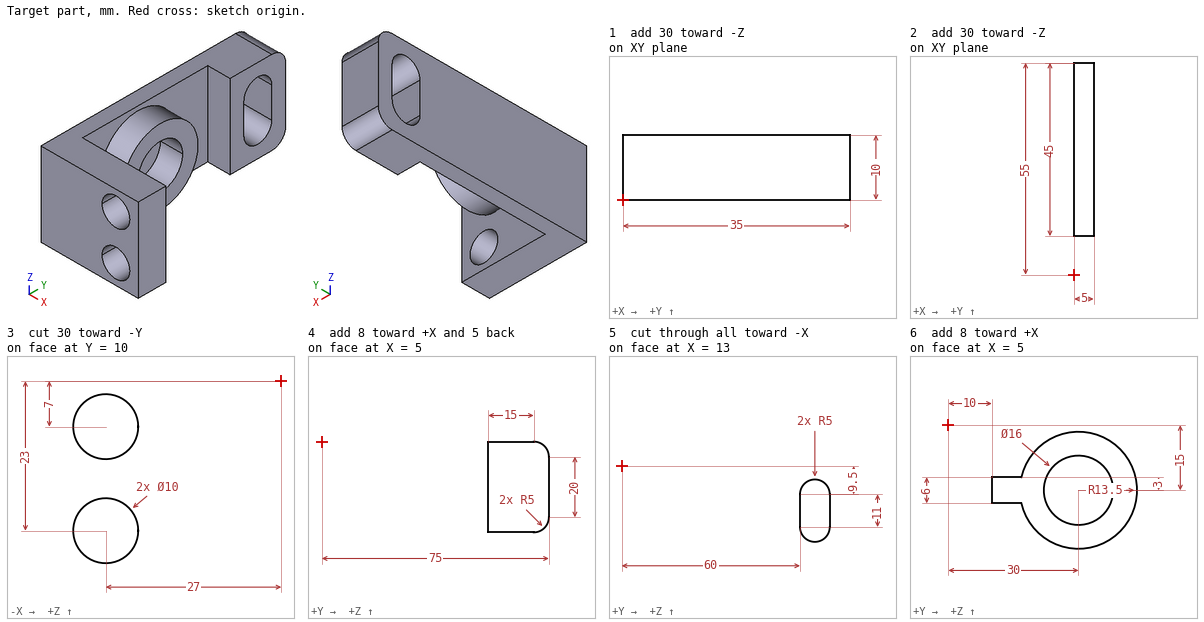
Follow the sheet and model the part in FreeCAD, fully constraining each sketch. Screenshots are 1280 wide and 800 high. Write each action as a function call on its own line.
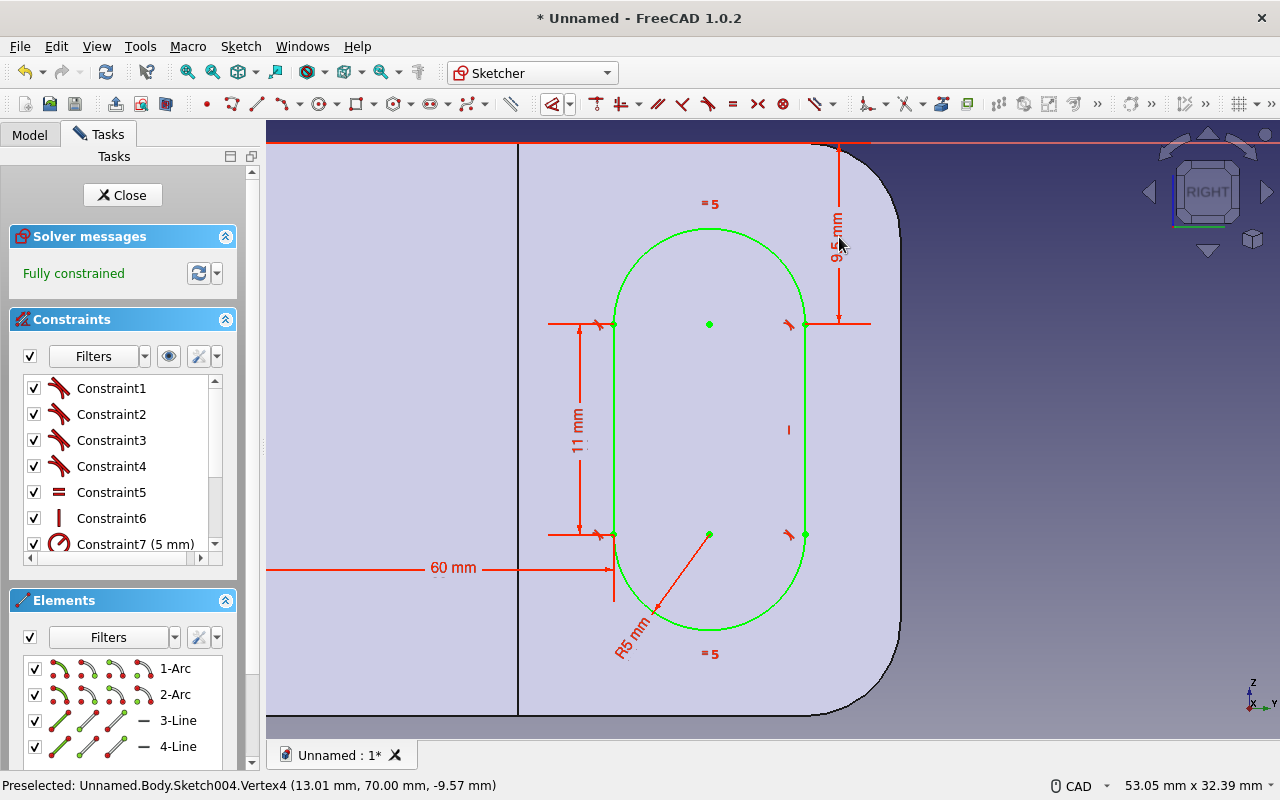
click(123, 195)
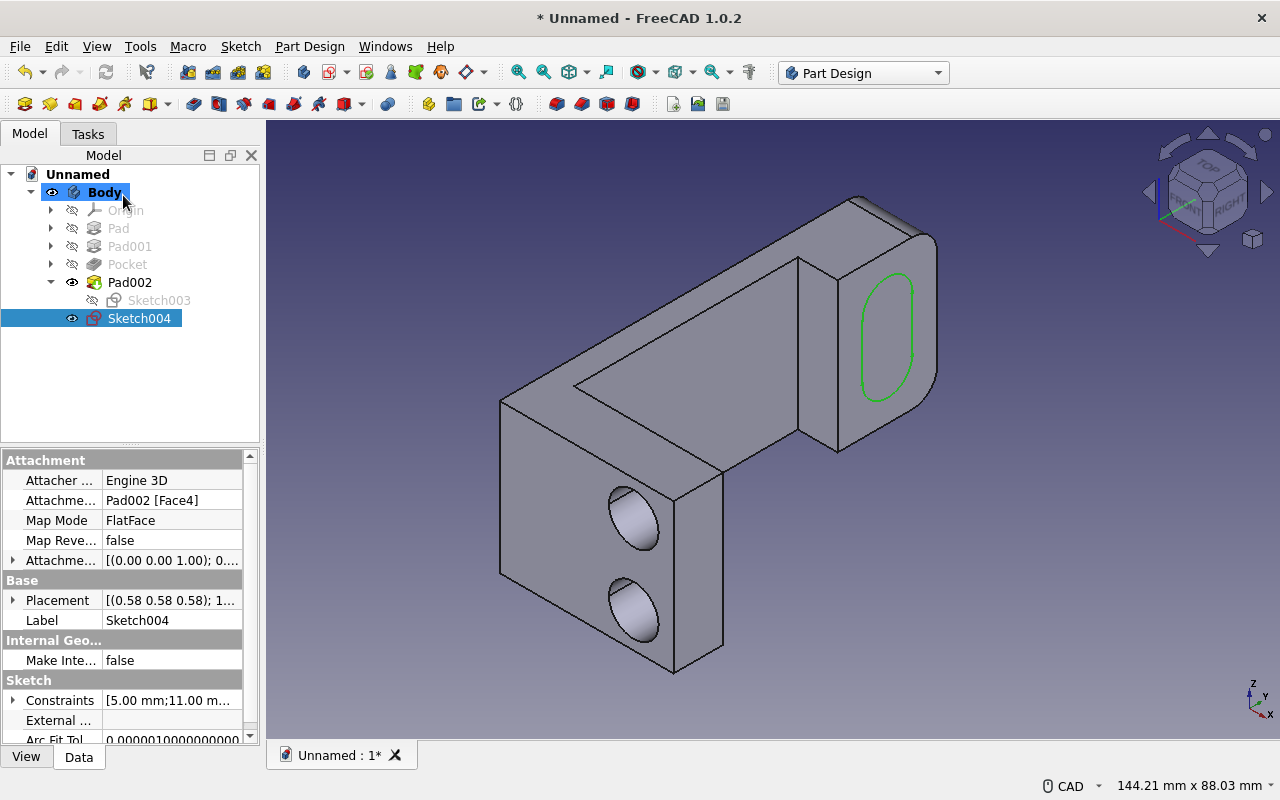
click(194, 104)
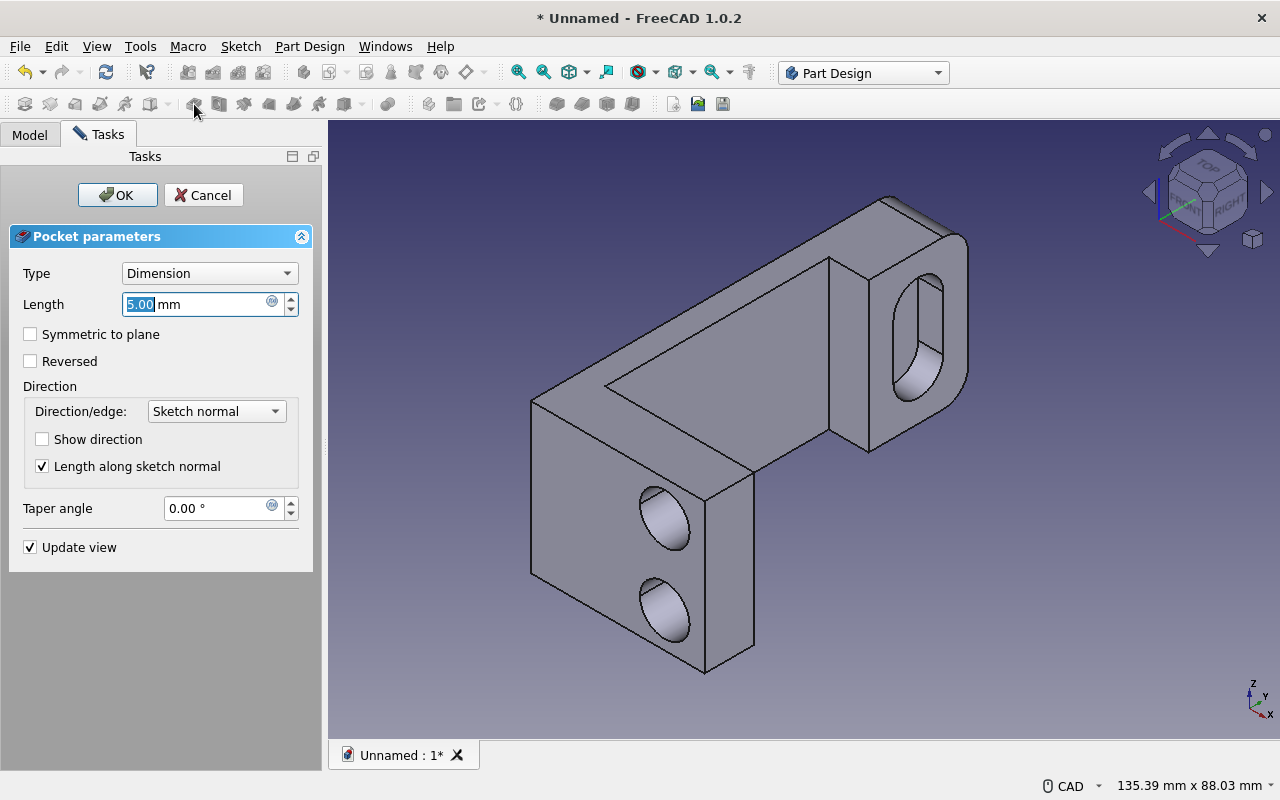
click(210, 274)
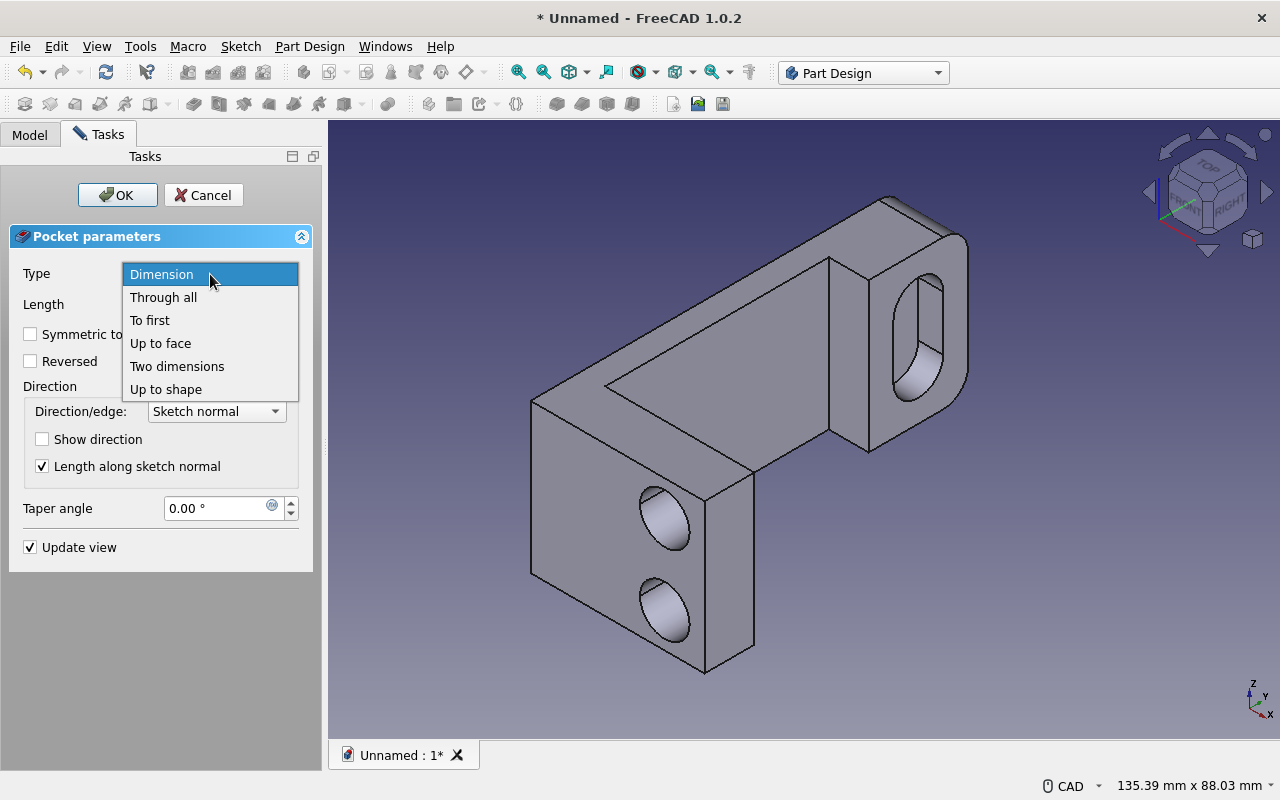
click(208, 298)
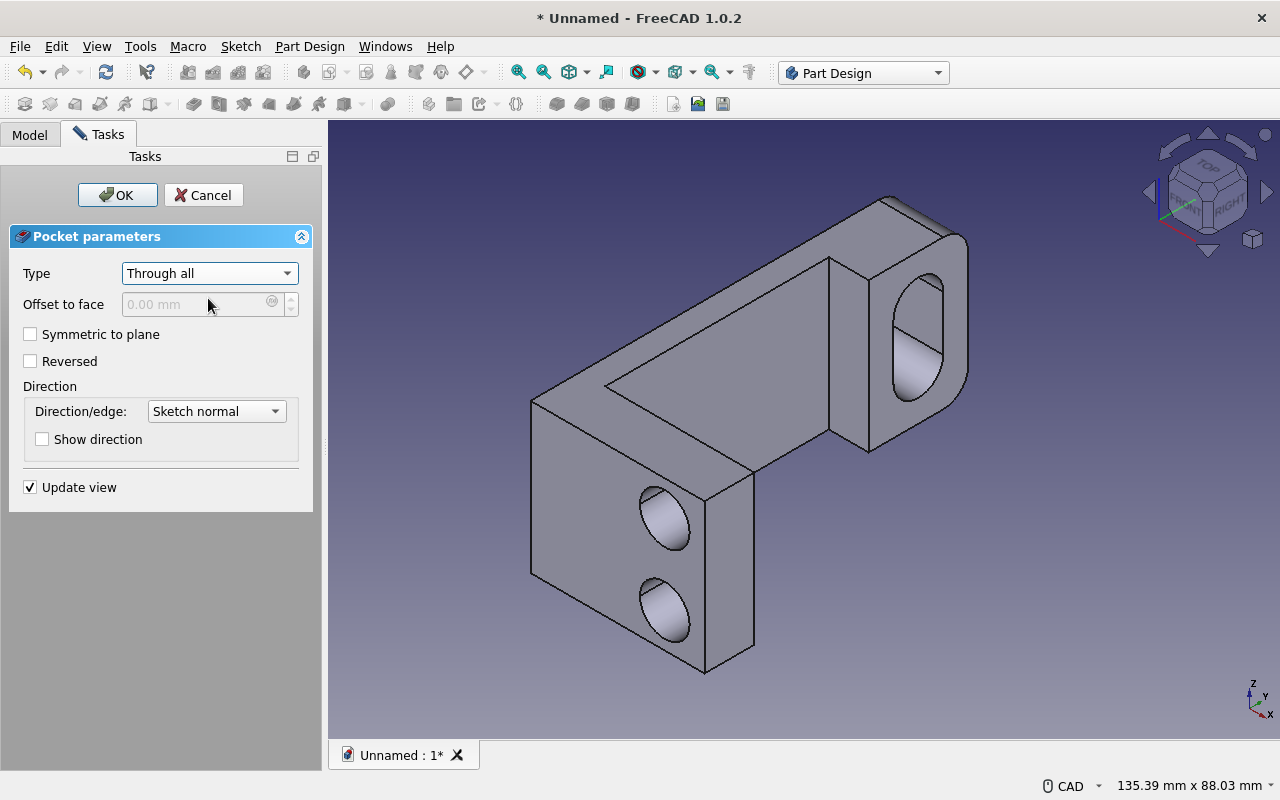
click(118, 195)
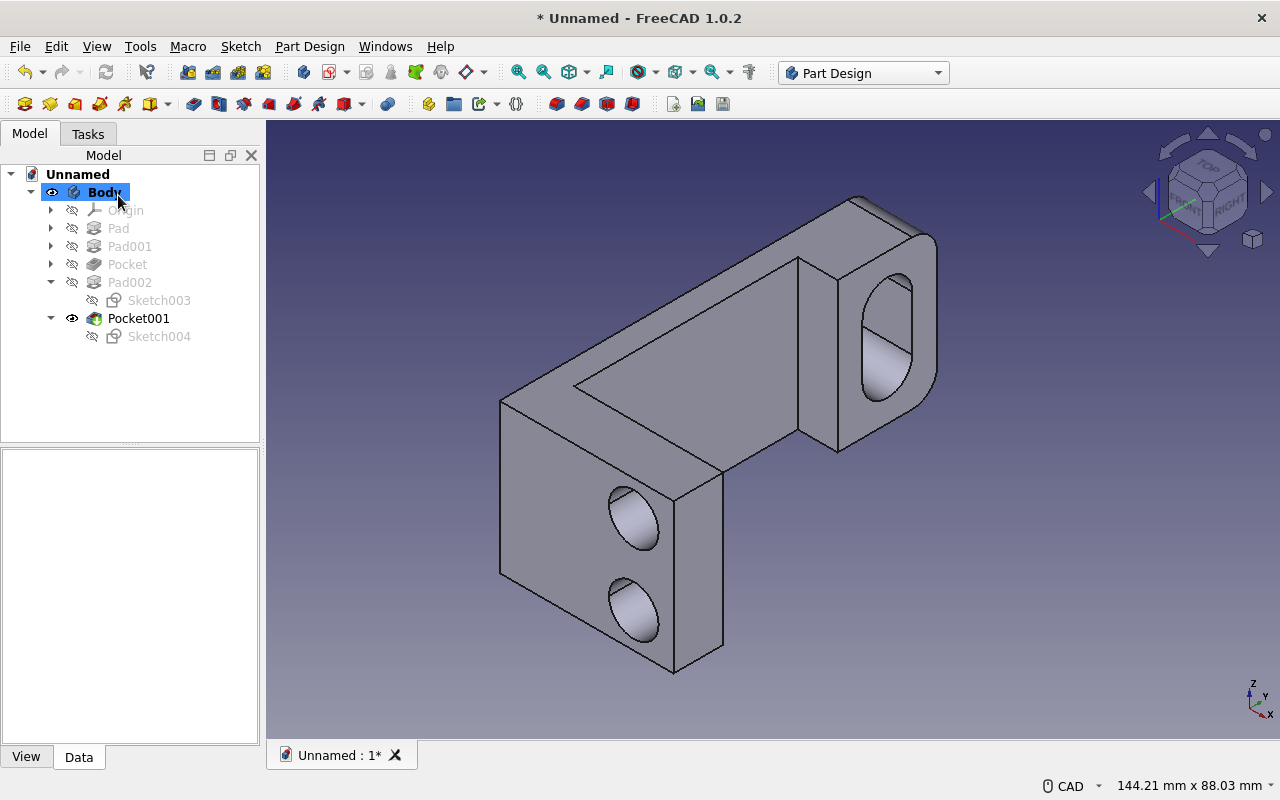
click(718, 389)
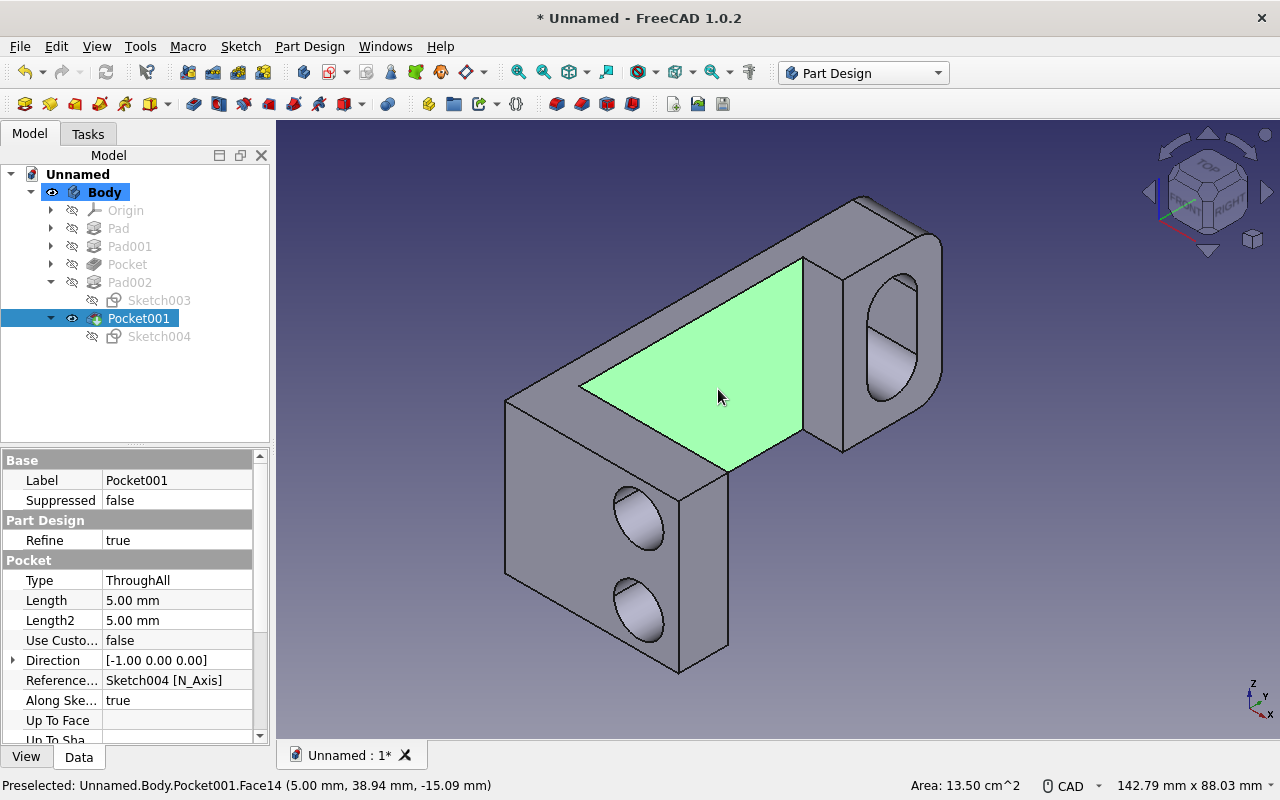
click(328, 72)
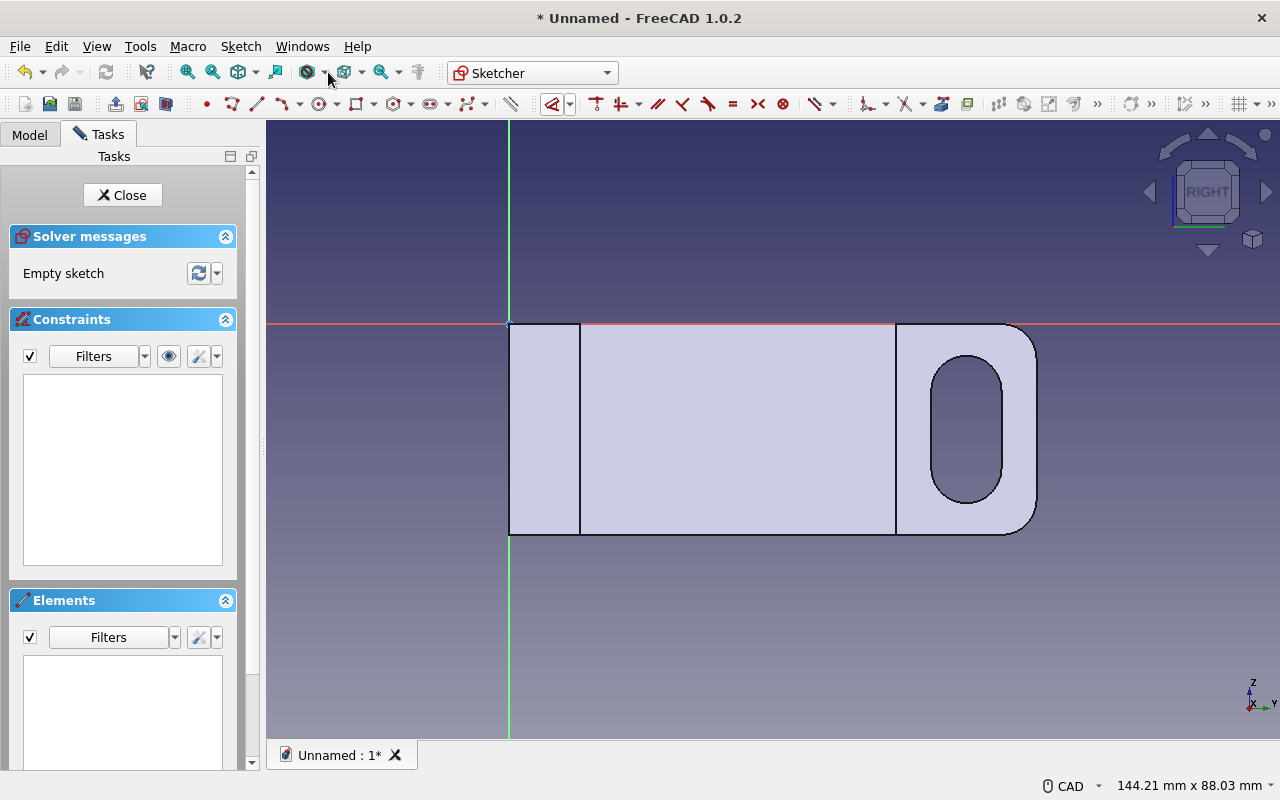
key(q)
key(s)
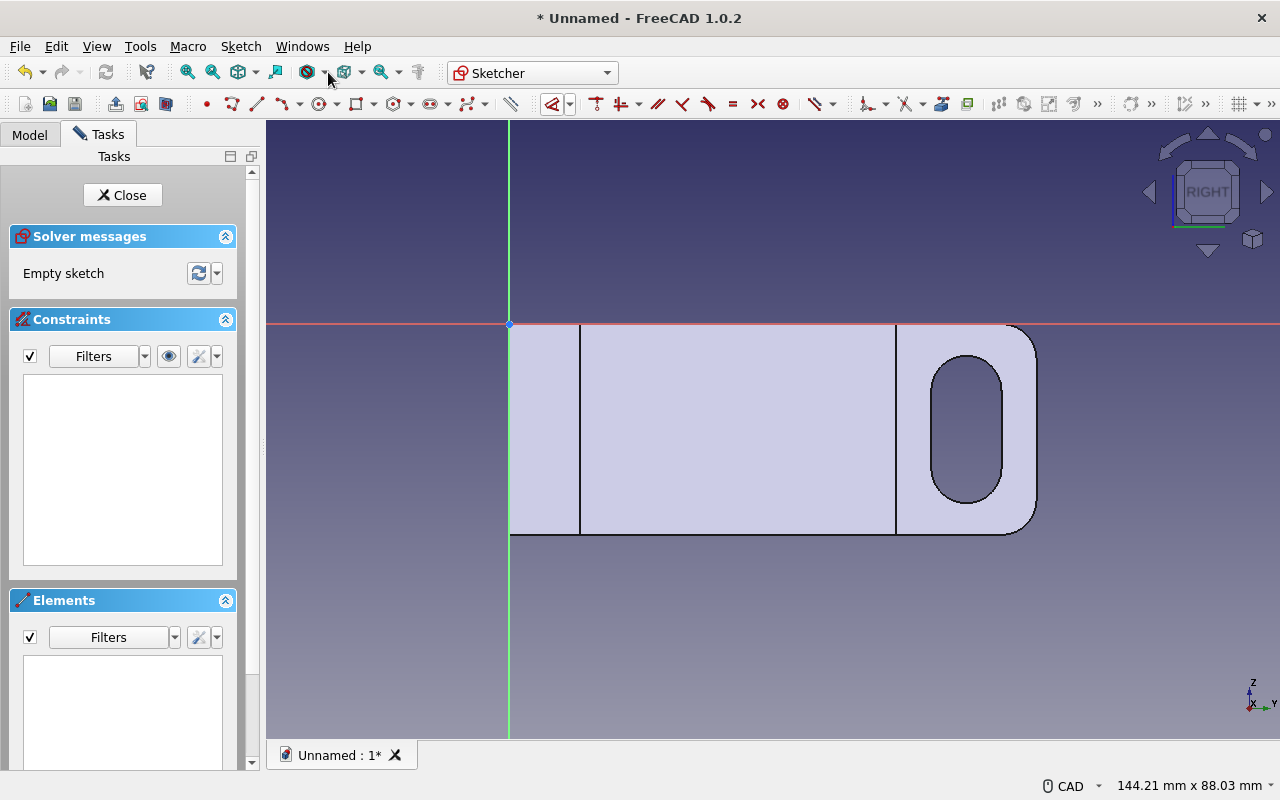
scroll(611, 375, up, 3)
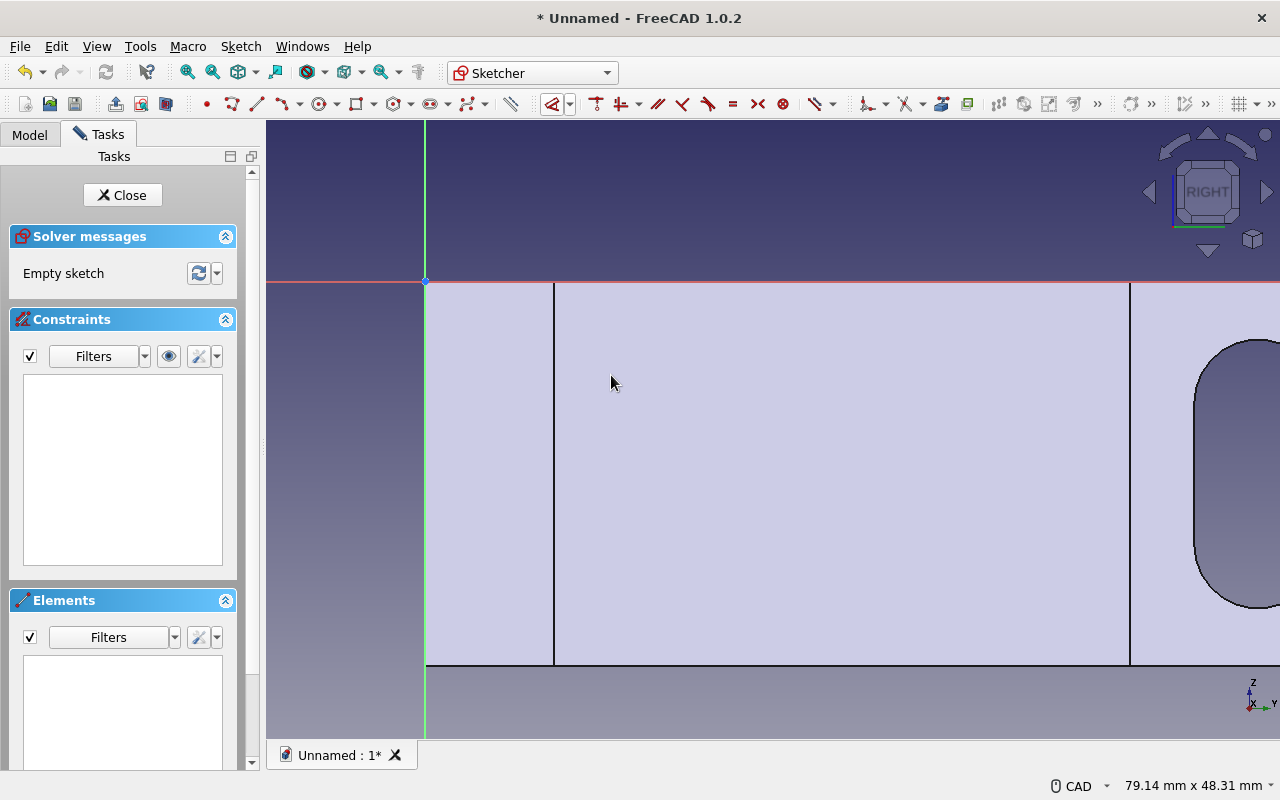
key(g)
key(m)